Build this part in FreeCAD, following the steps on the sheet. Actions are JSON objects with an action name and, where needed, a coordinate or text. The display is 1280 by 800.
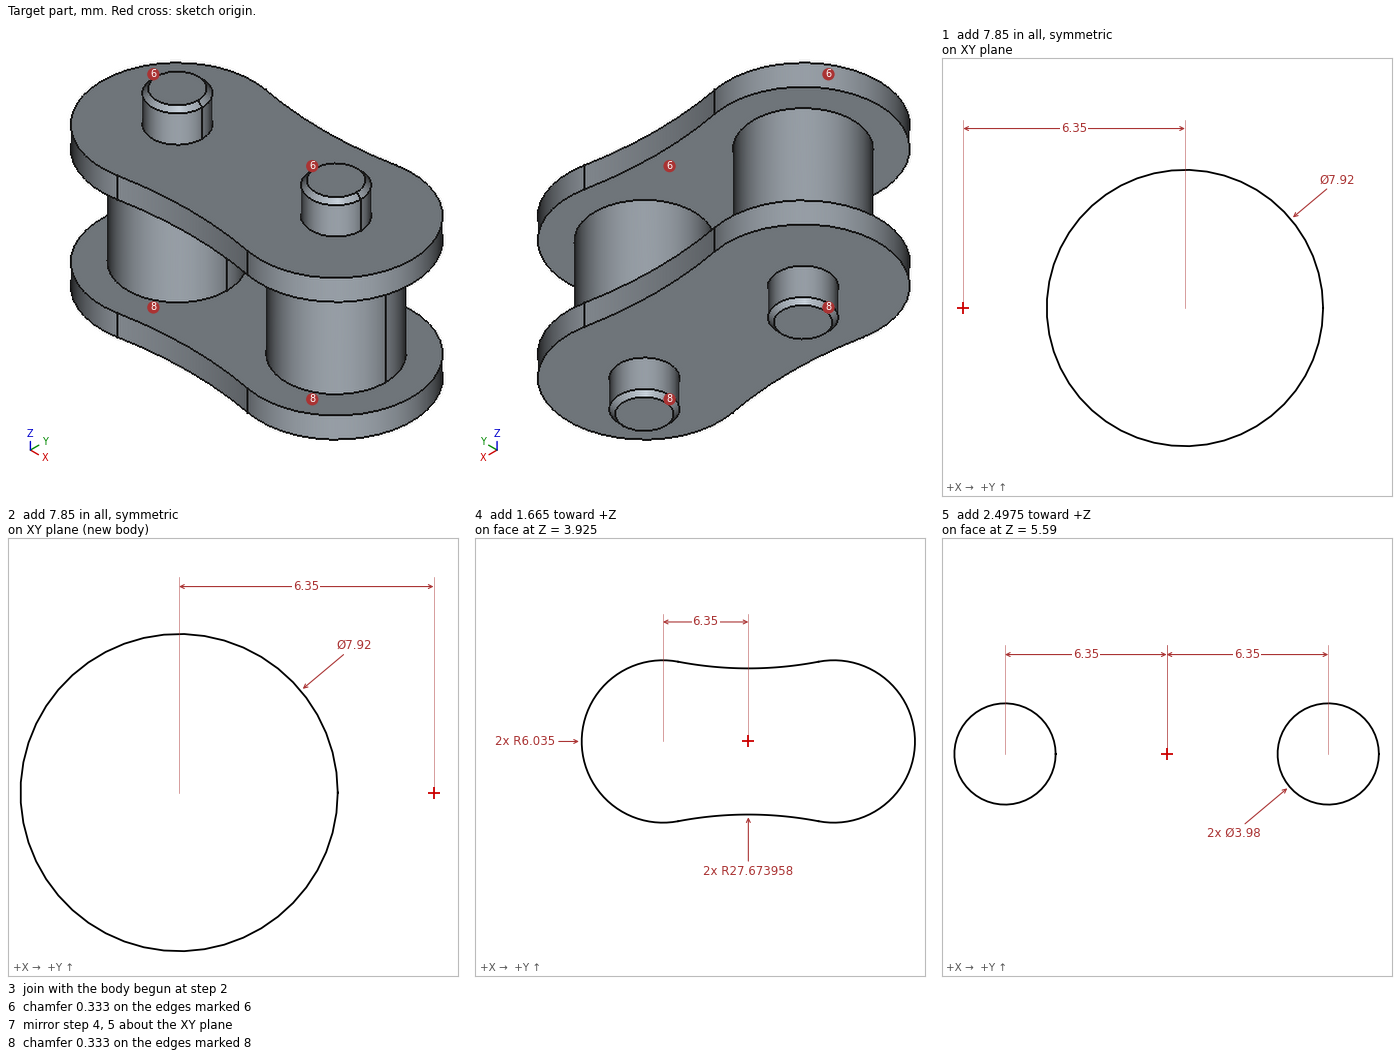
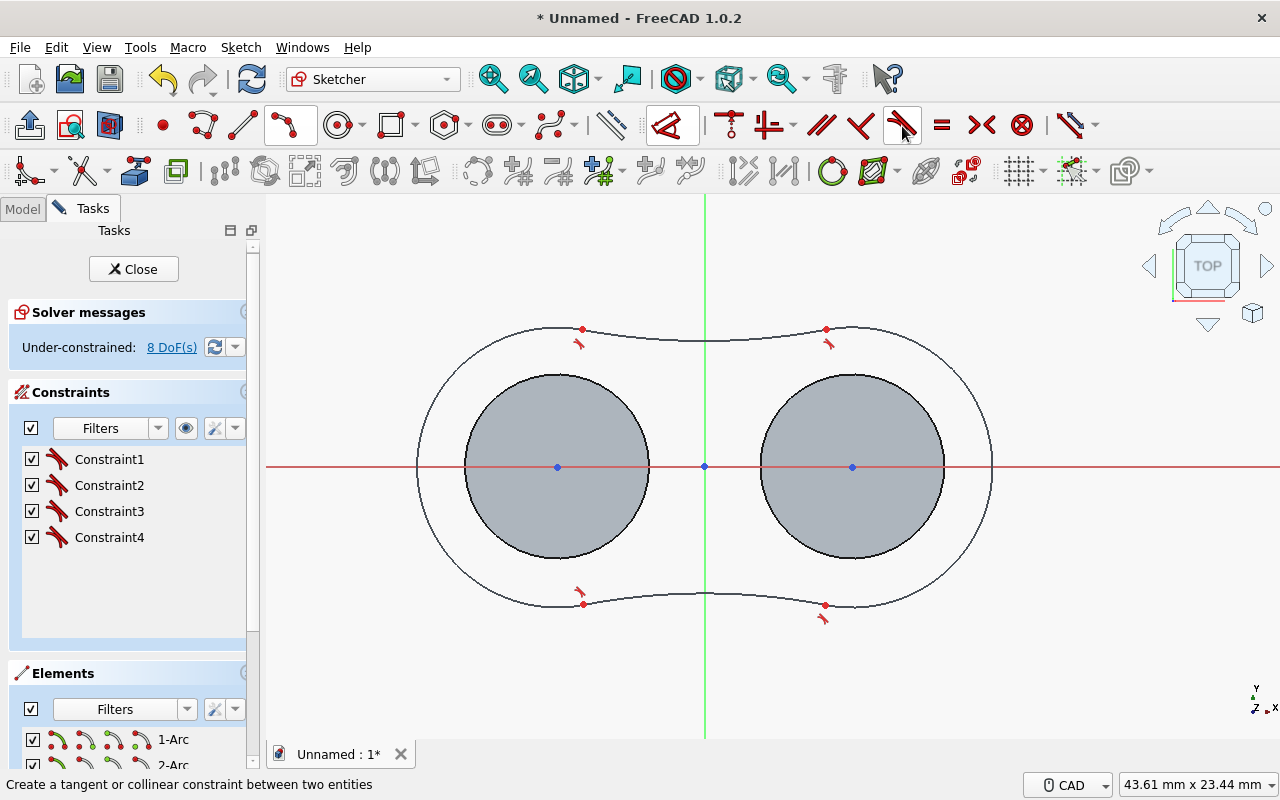
{"action": "left_click", "coordinate": [450, 378]}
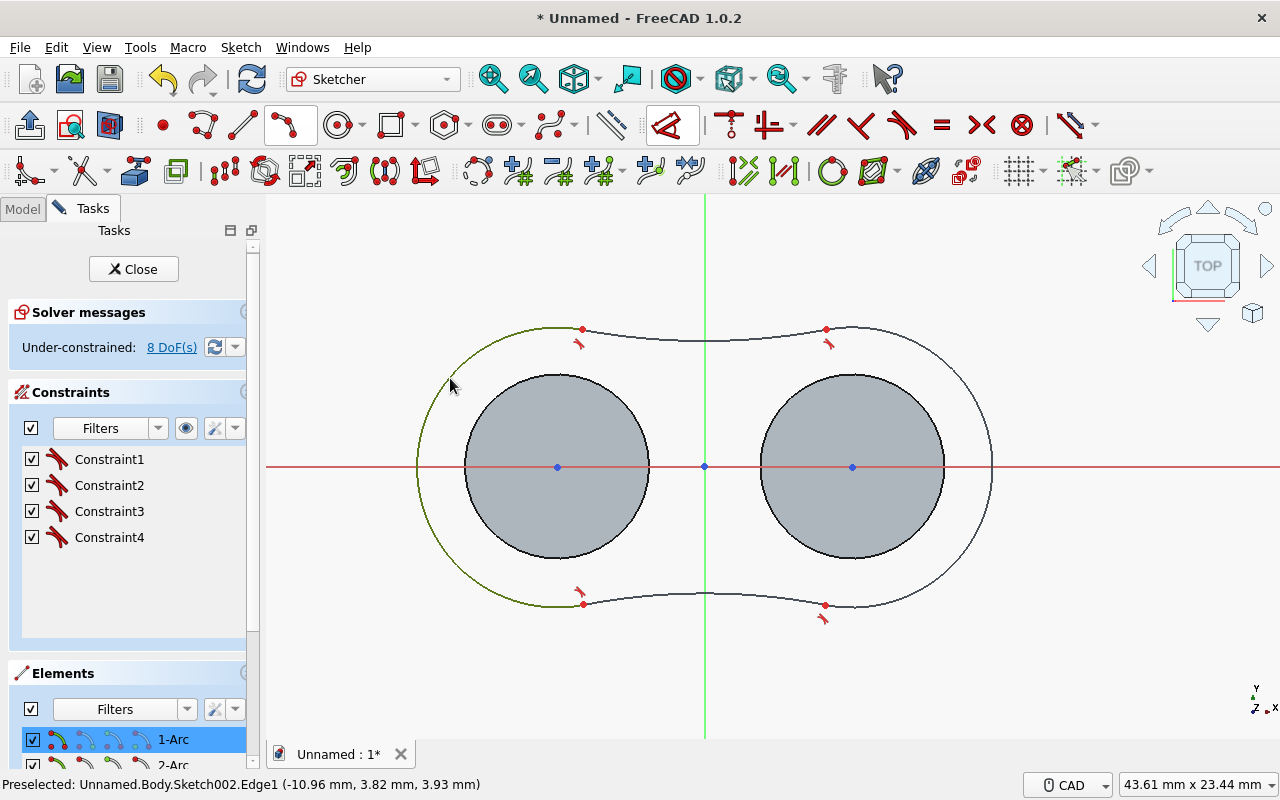
{"action": "left_click", "coordinate": [959, 558]}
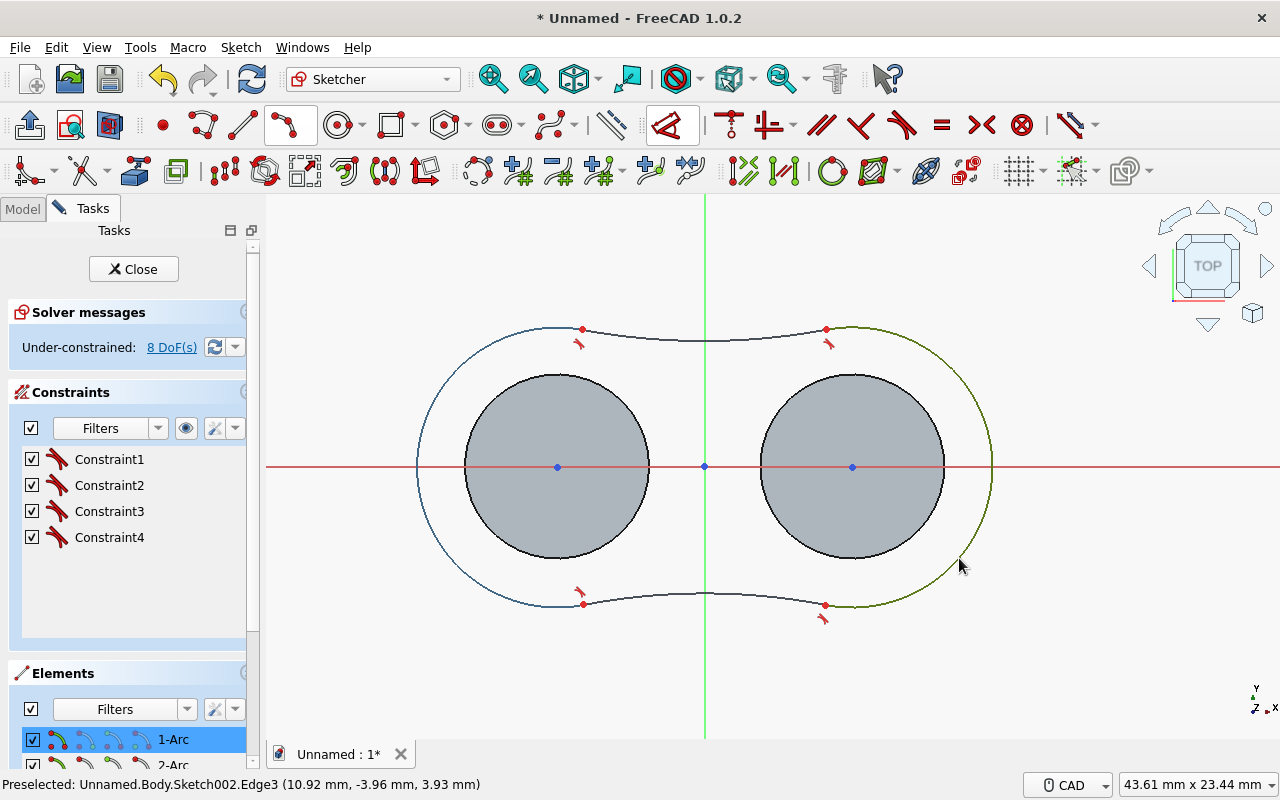
{"action": "left_click", "coordinate": [942, 126]}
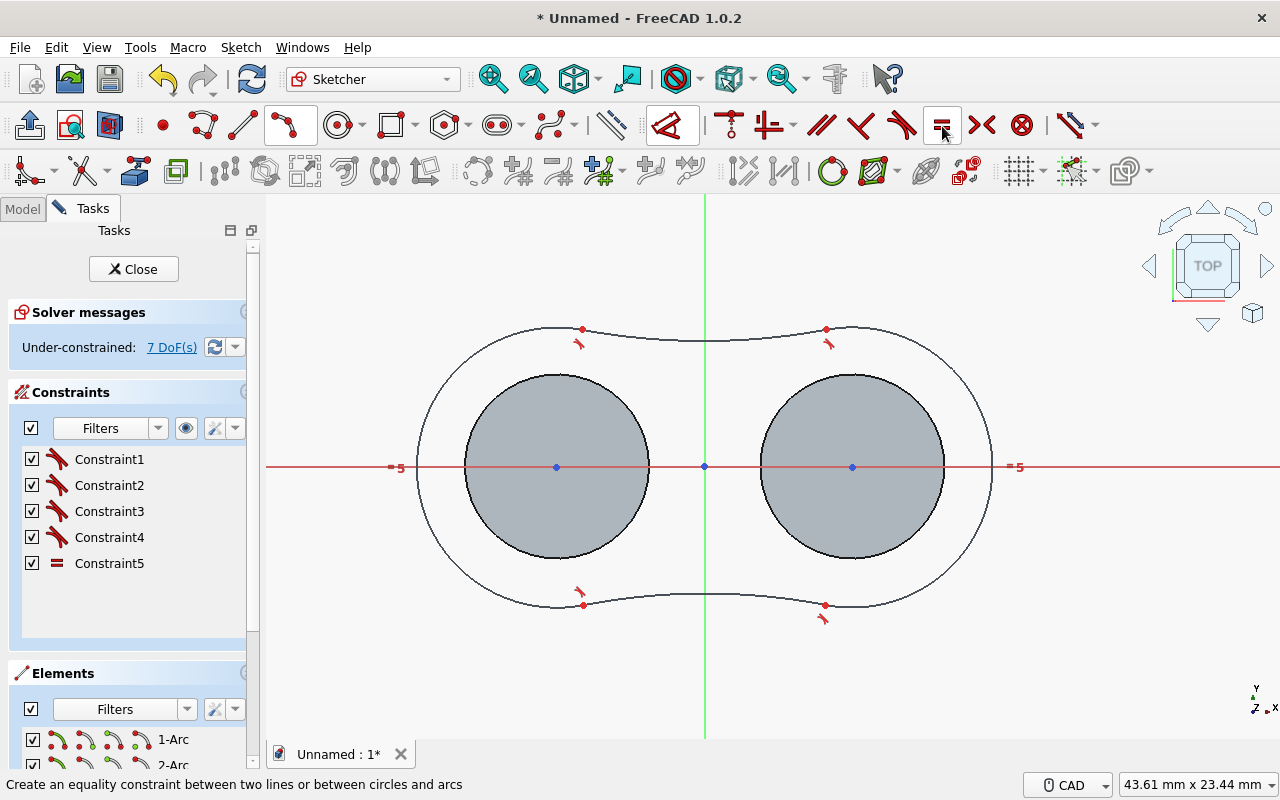
{"action": "left_click", "coordinate": [753, 595]}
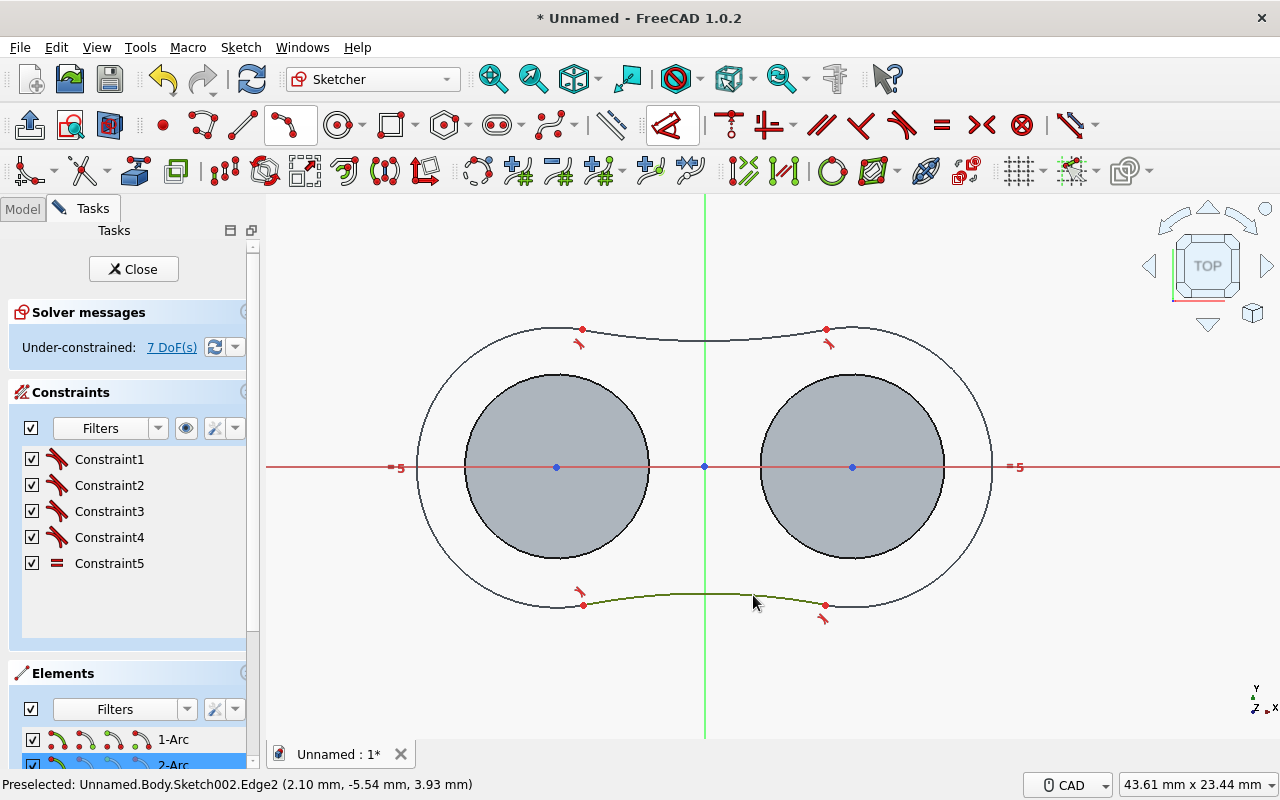
{"action": "left_click", "coordinate": [655, 339]}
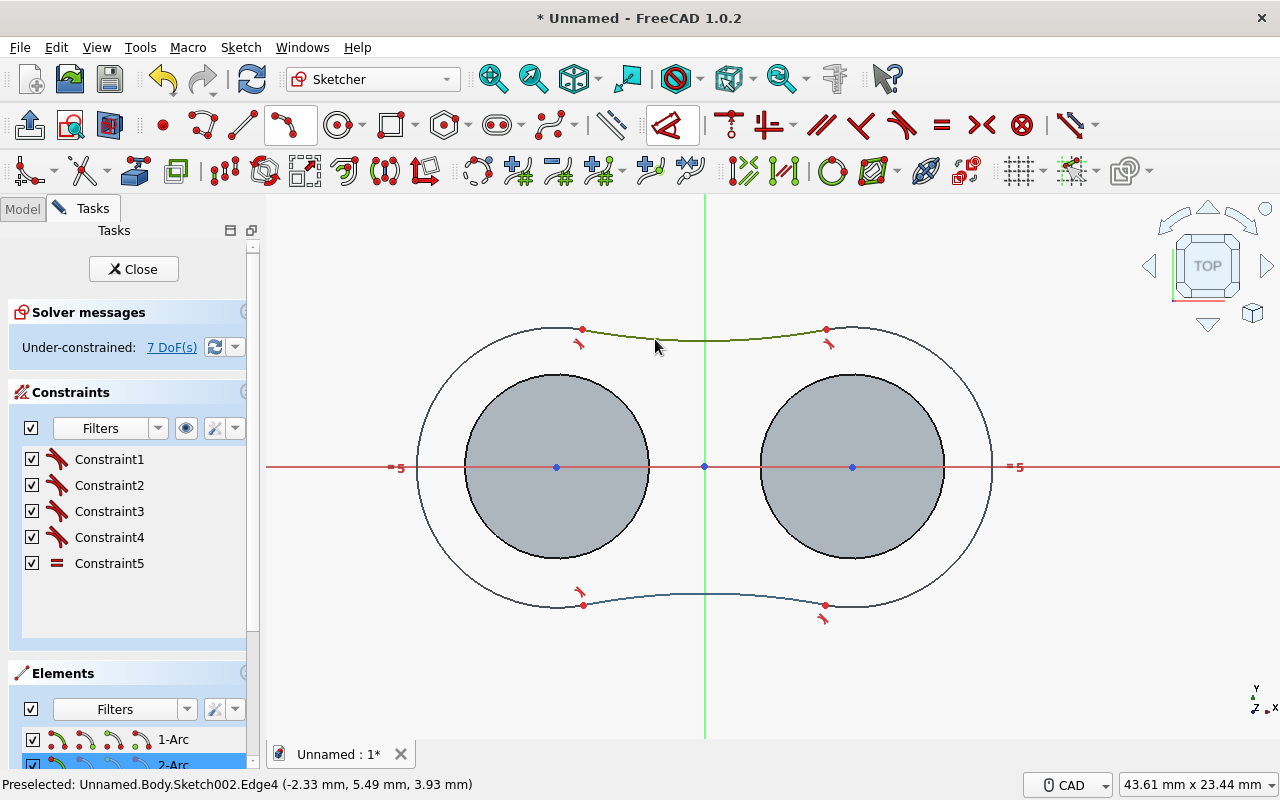
{"action": "key", "text": "e"}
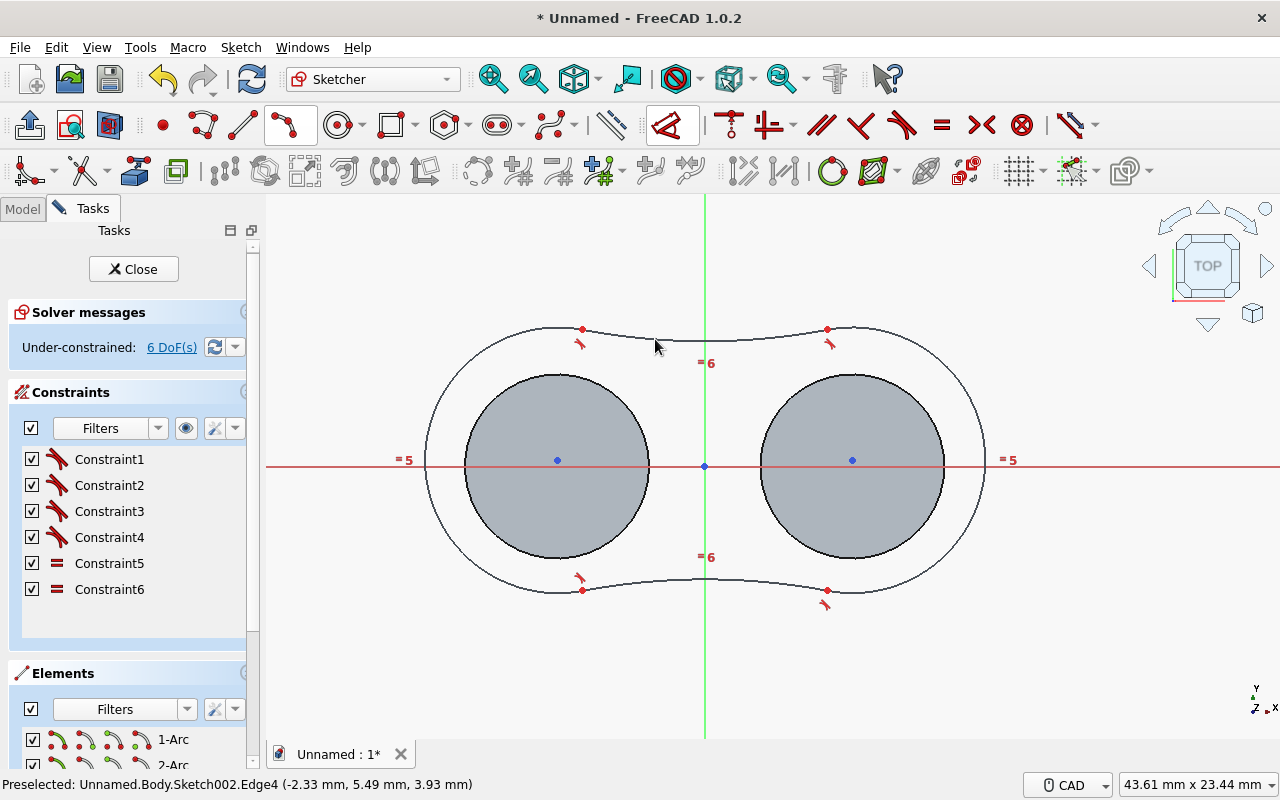
{"action": "left_click", "coordinate": [558, 460]}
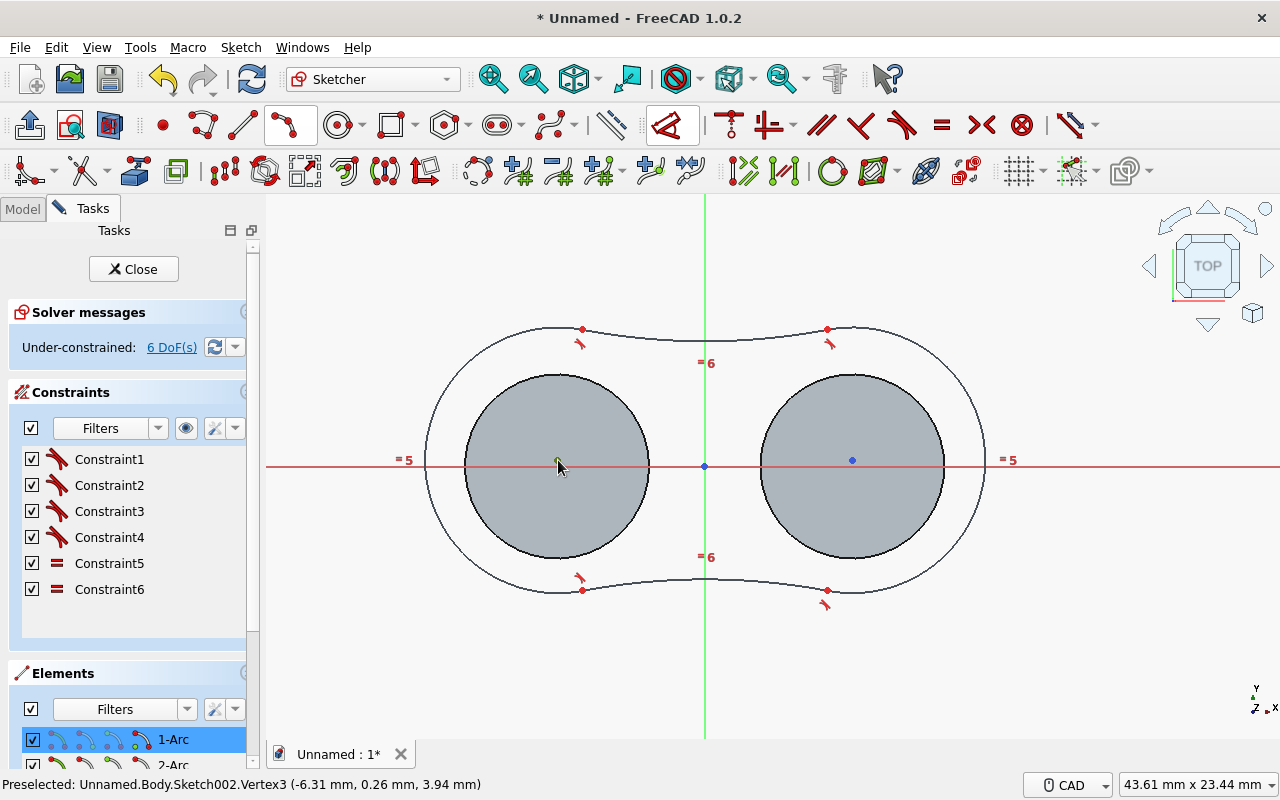
{"action": "left_click", "coordinate": [353, 466]}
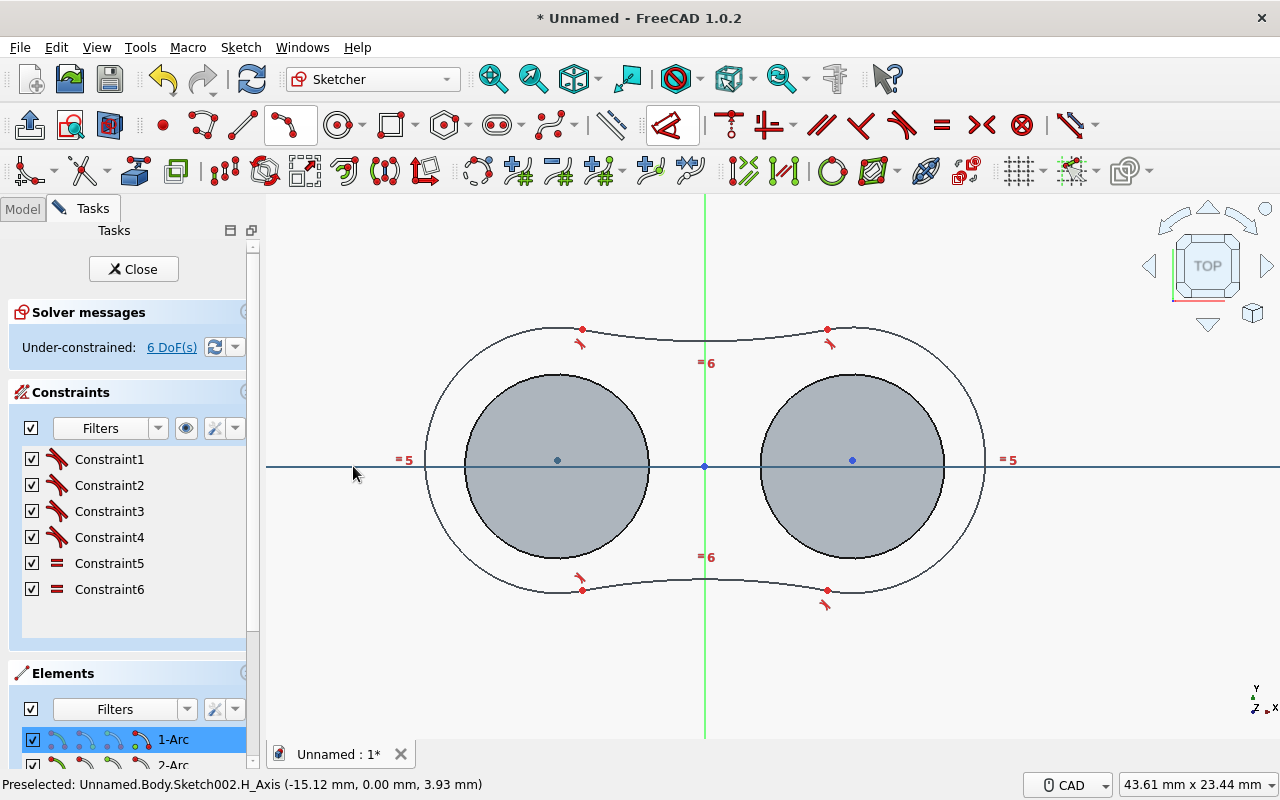
{"action": "left_click", "coordinate": [730, 126]}